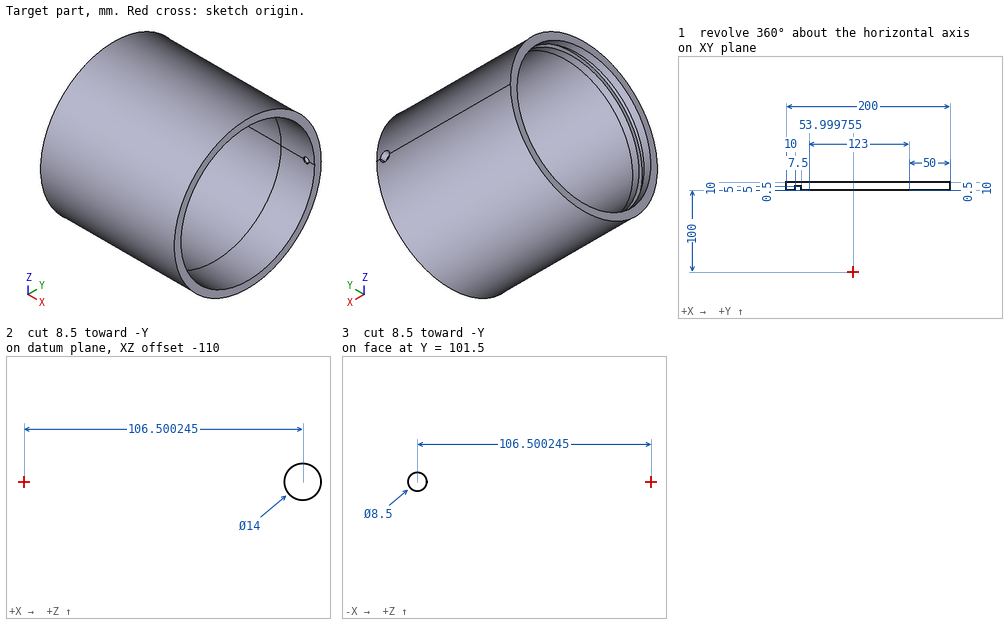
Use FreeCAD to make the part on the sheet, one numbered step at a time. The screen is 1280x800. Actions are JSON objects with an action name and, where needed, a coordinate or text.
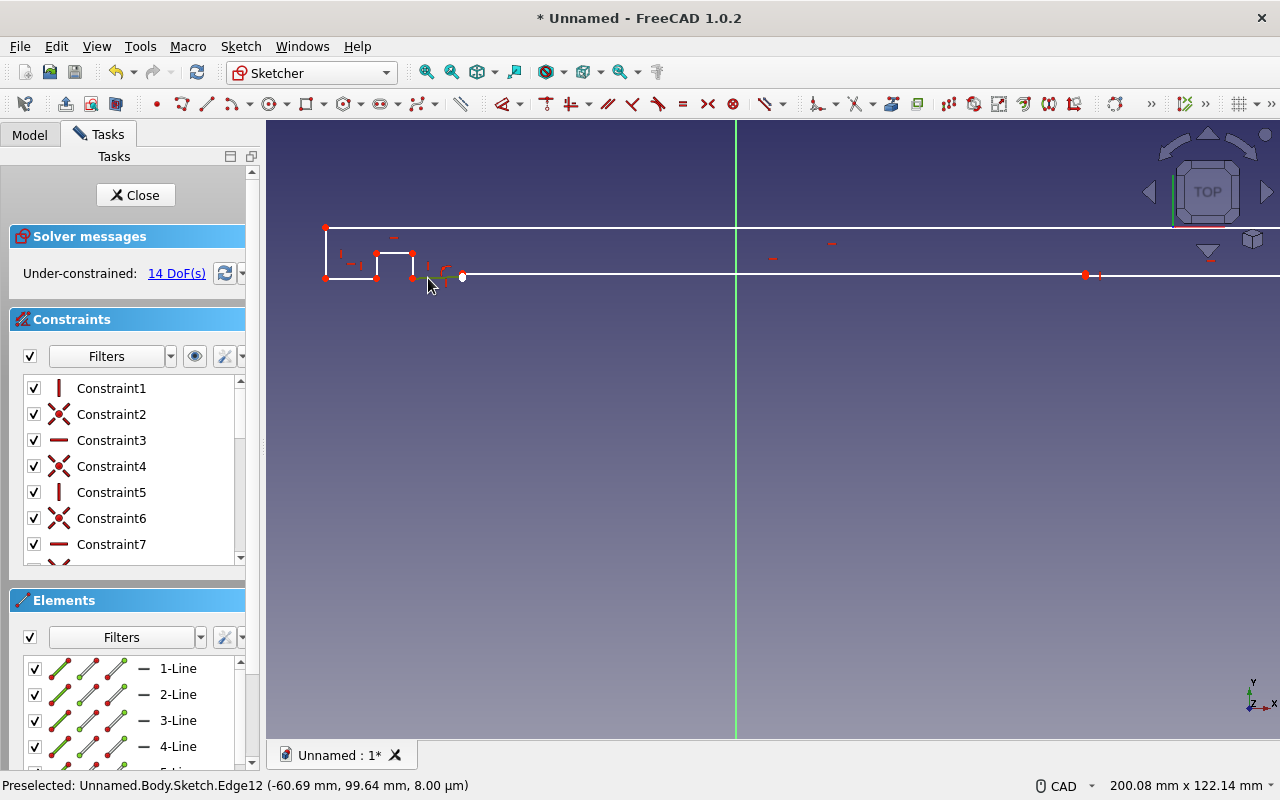
{"action": "key", "text": "h"}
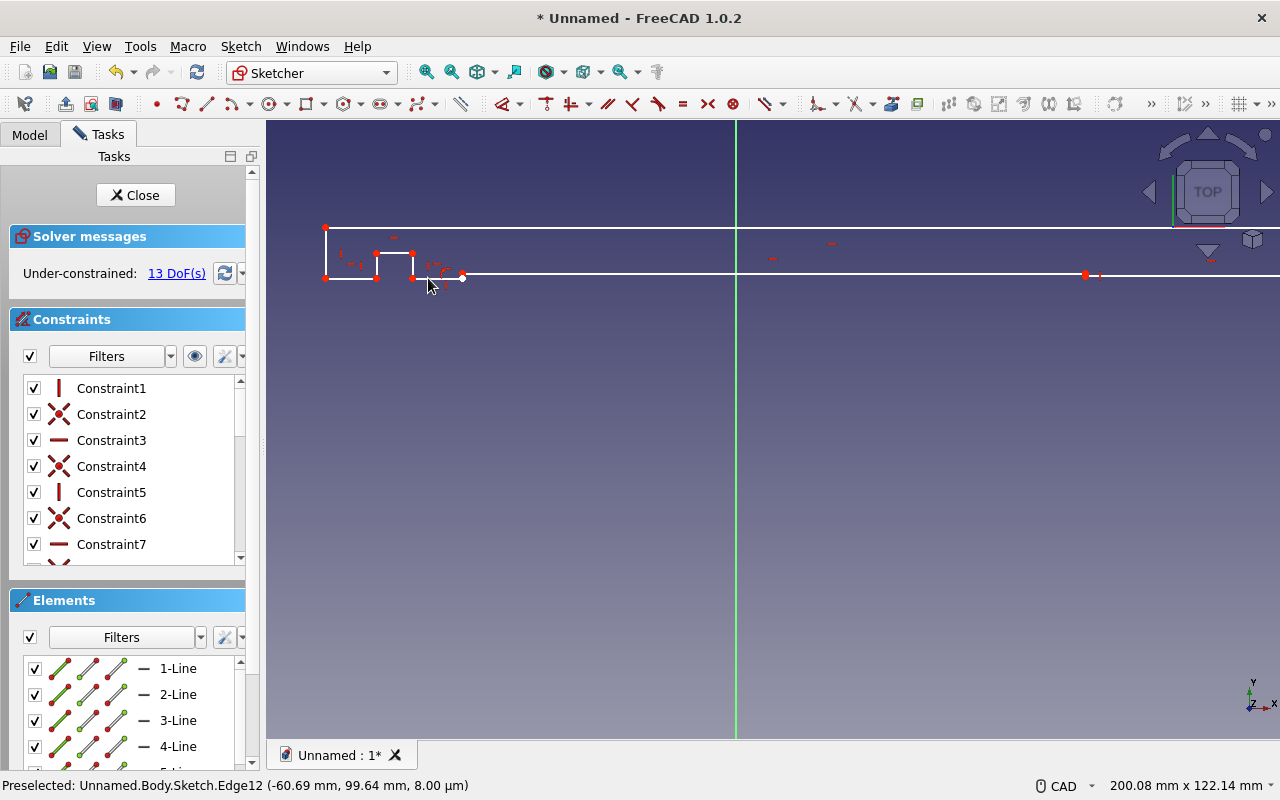
{"action": "left_click", "coordinate": [502, 104]}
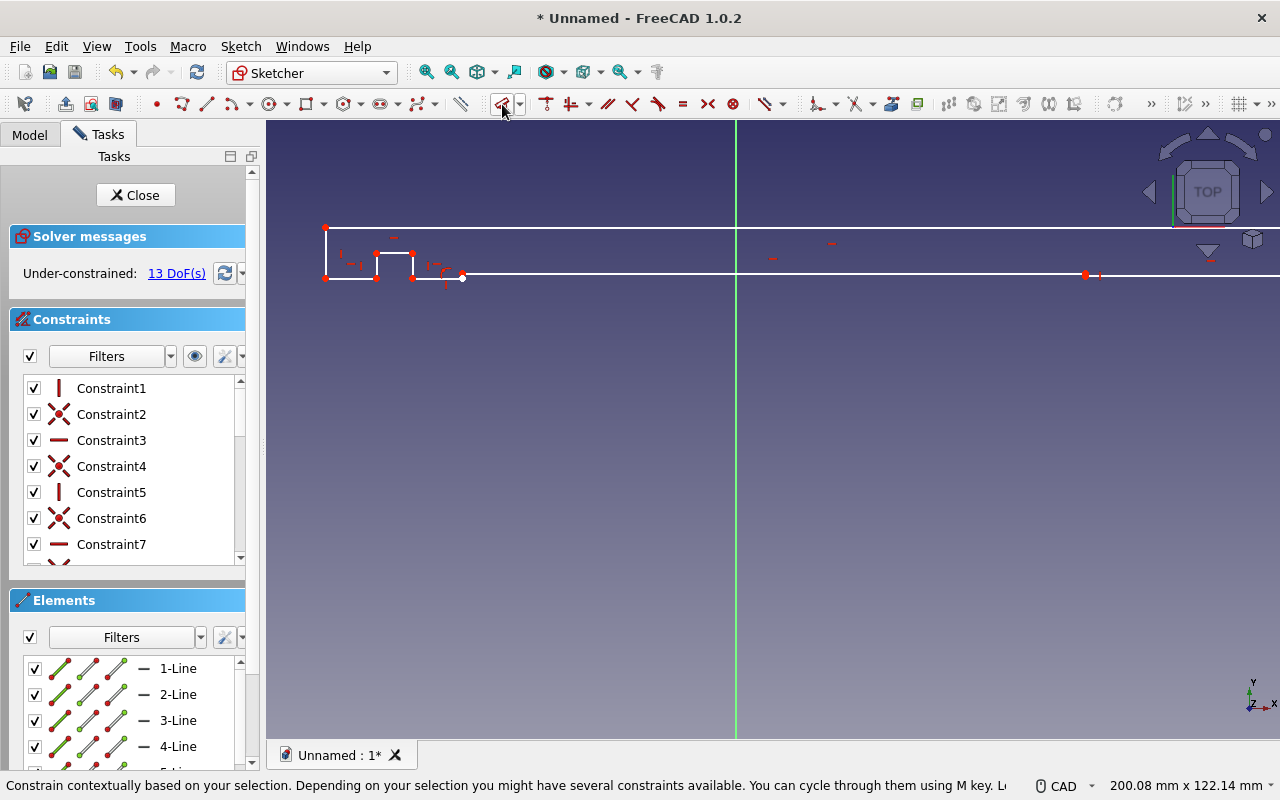
{"action": "scroll", "coordinate": [377, 268], "scroll_direction": "up", "scroll_amount": 3}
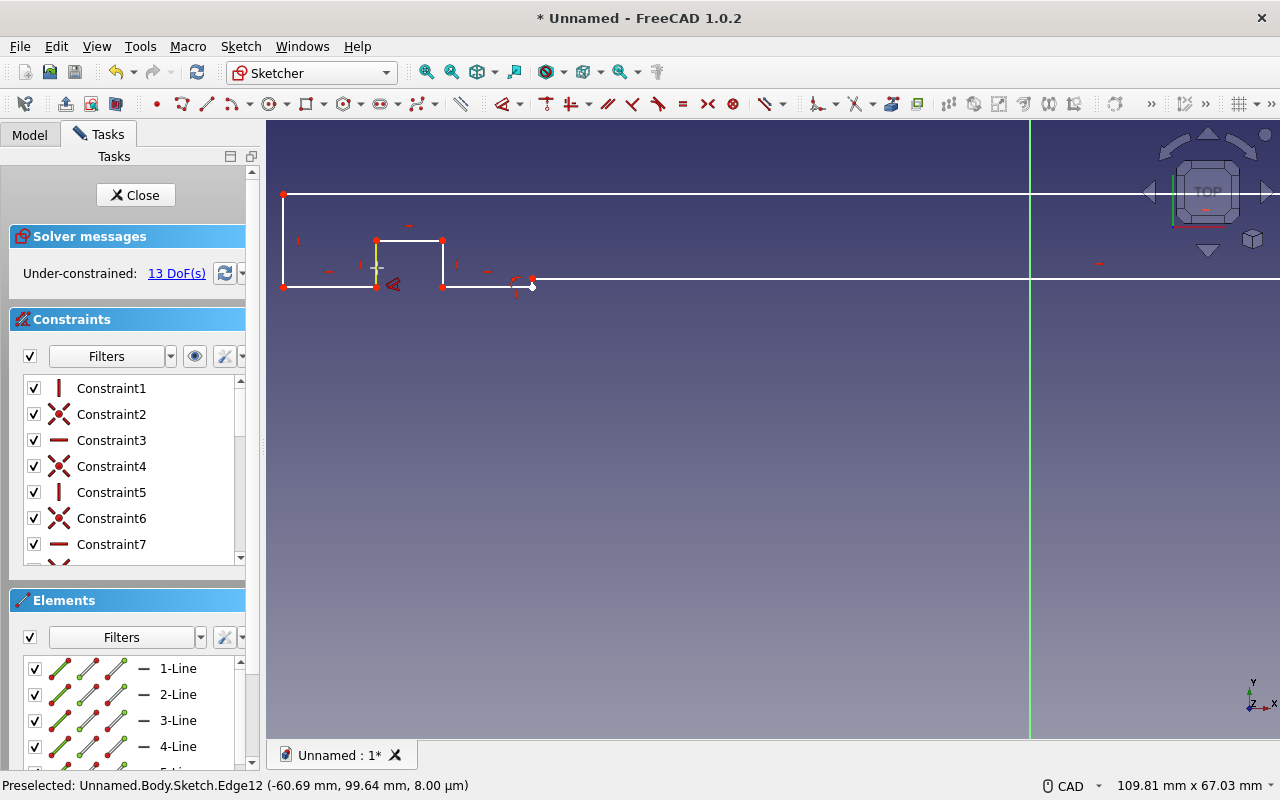
{"action": "left_click", "coordinate": [376, 269]}
{"action": "left_click", "coordinate": [342, 264]}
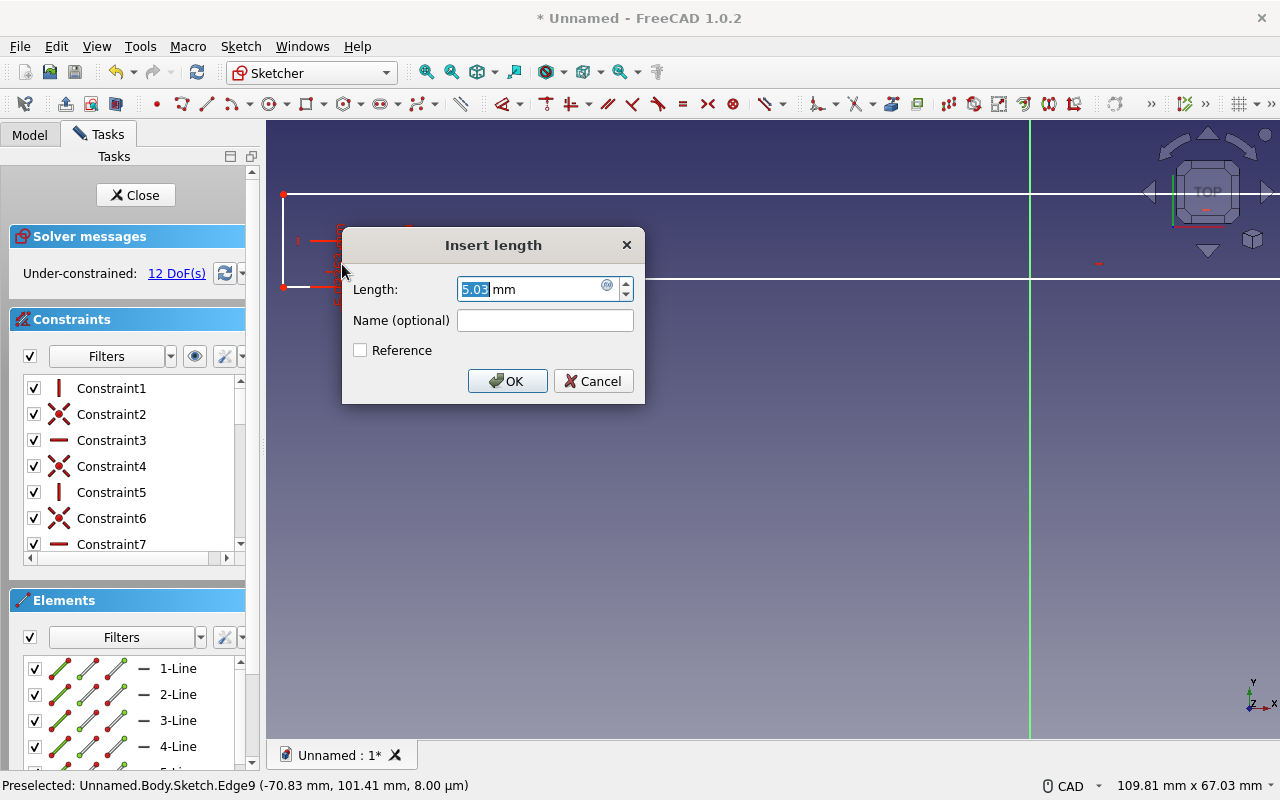
{"action": "type", "text": "5"}
{"action": "key", "text": "Return"}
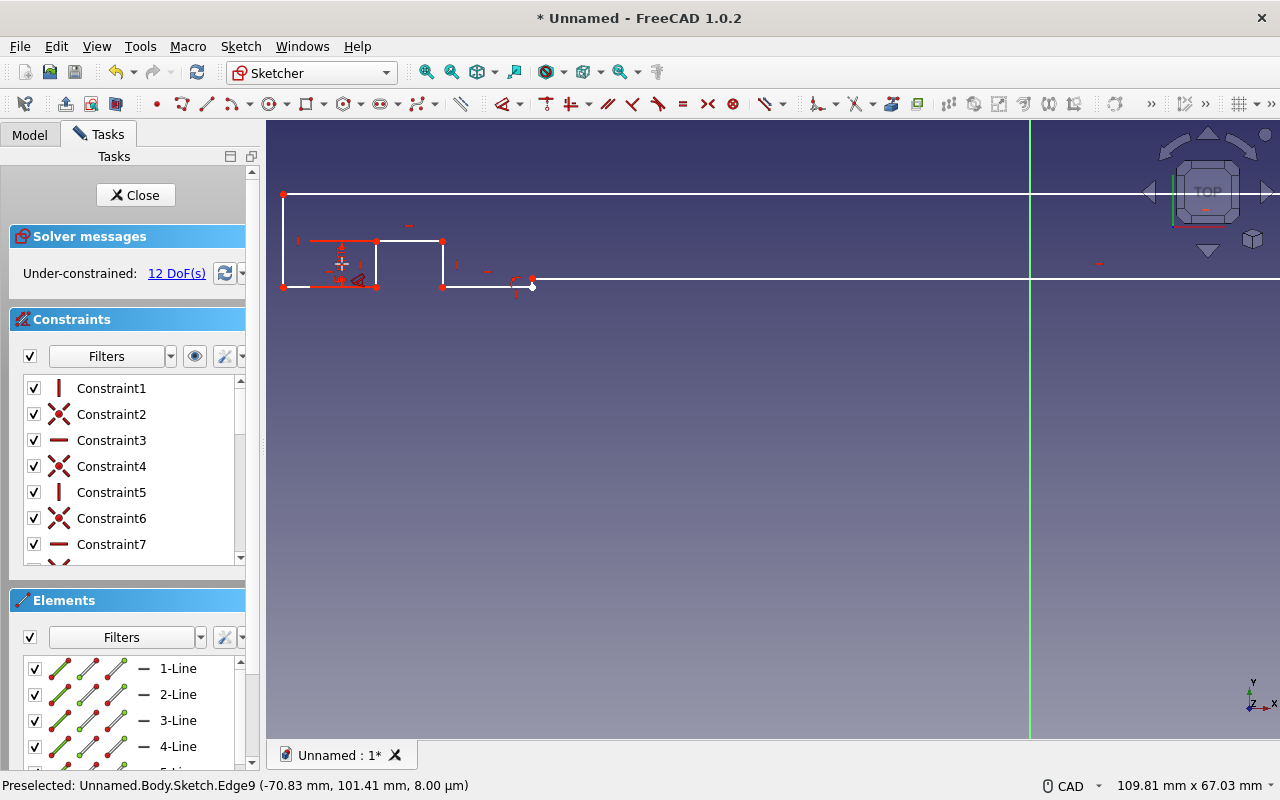
{"action": "left_click", "coordinate": [443, 255]}
{"action": "left_click", "coordinate": [477, 264]}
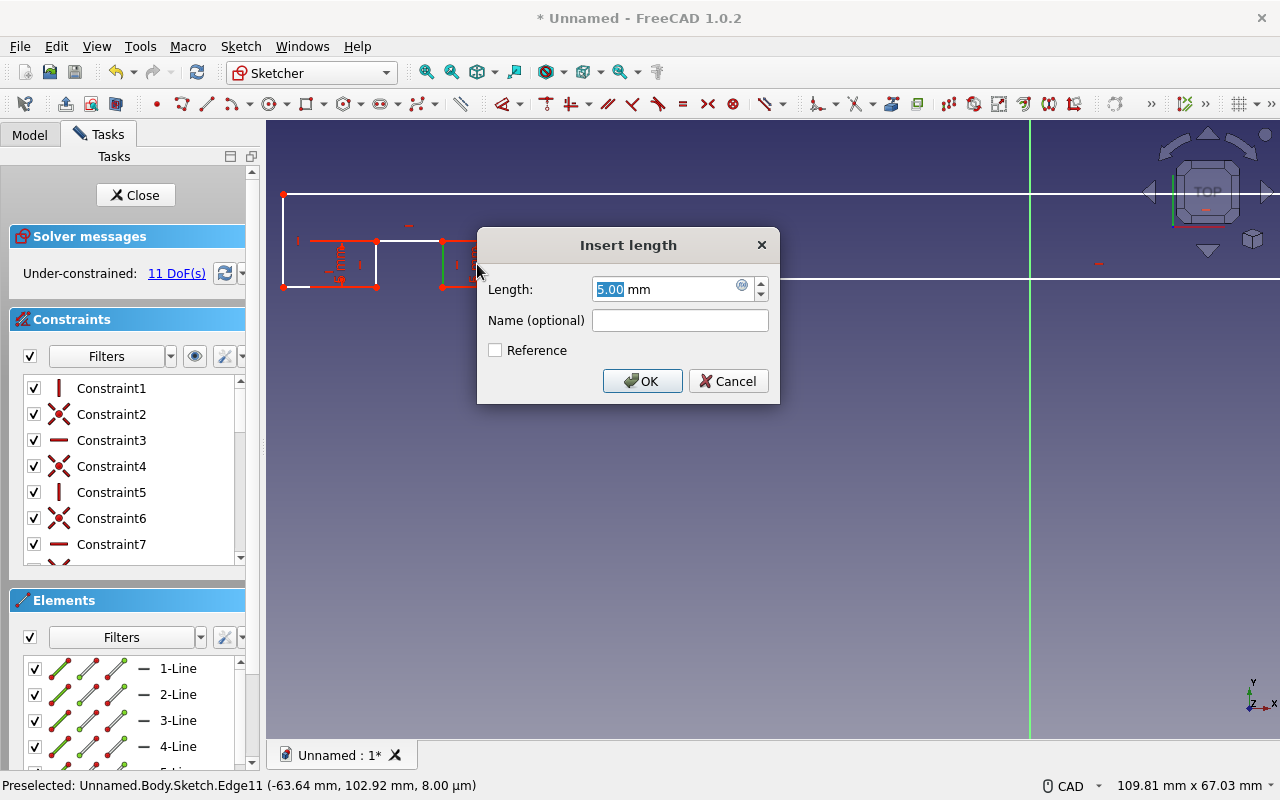
{"action": "type", "text": "5"}
{"action": "key", "text": "Return"}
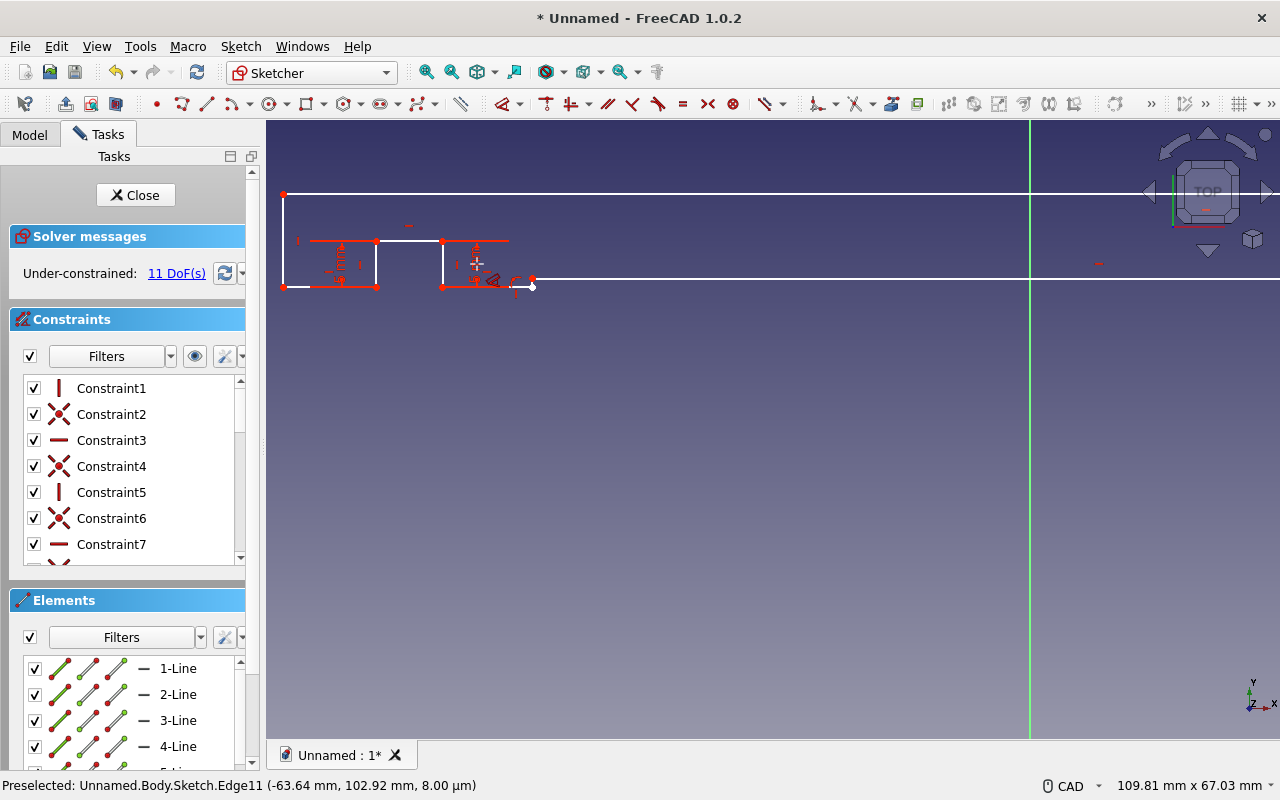
{"action": "scroll", "coordinate": [488, 314], "scroll_direction": "down", "scroll_amount": 6}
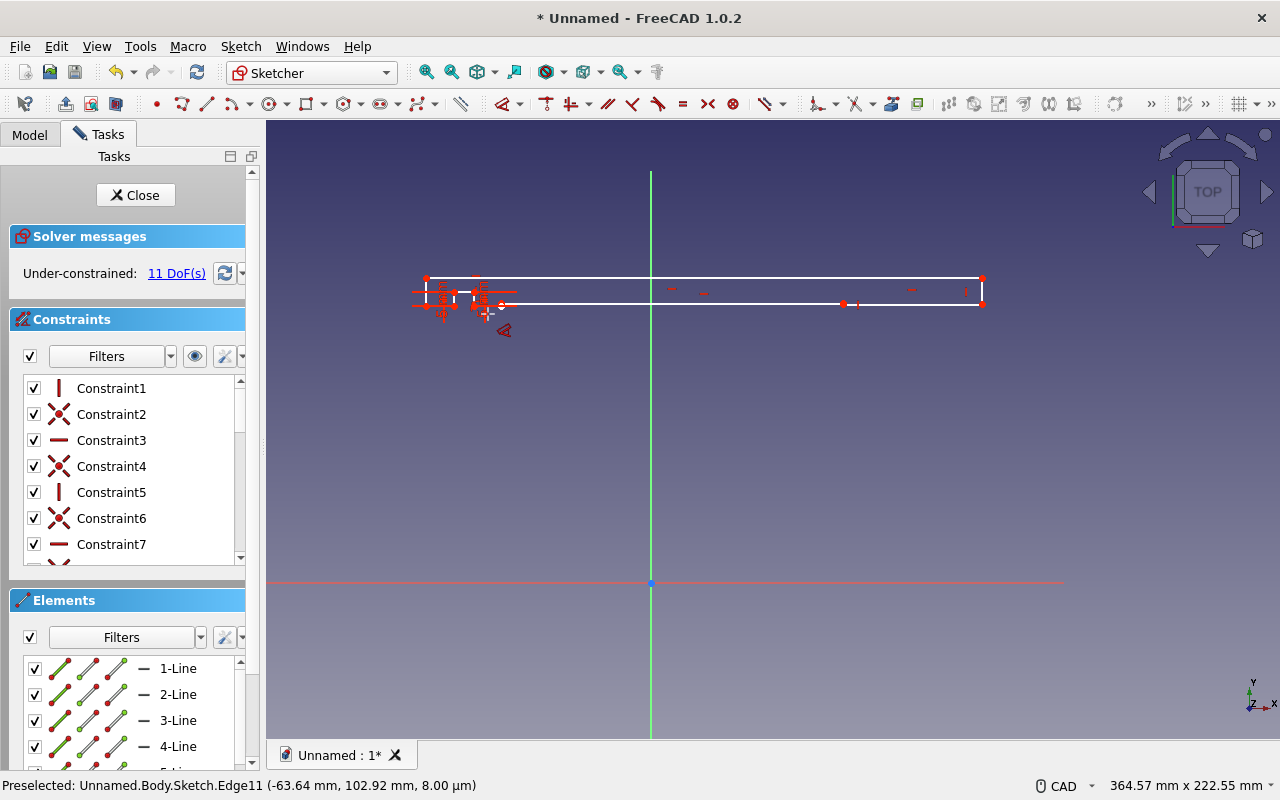
{"action": "left_click", "coordinate": [885, 305]}
{"action": "left_click", "coordinate": [913, 339]}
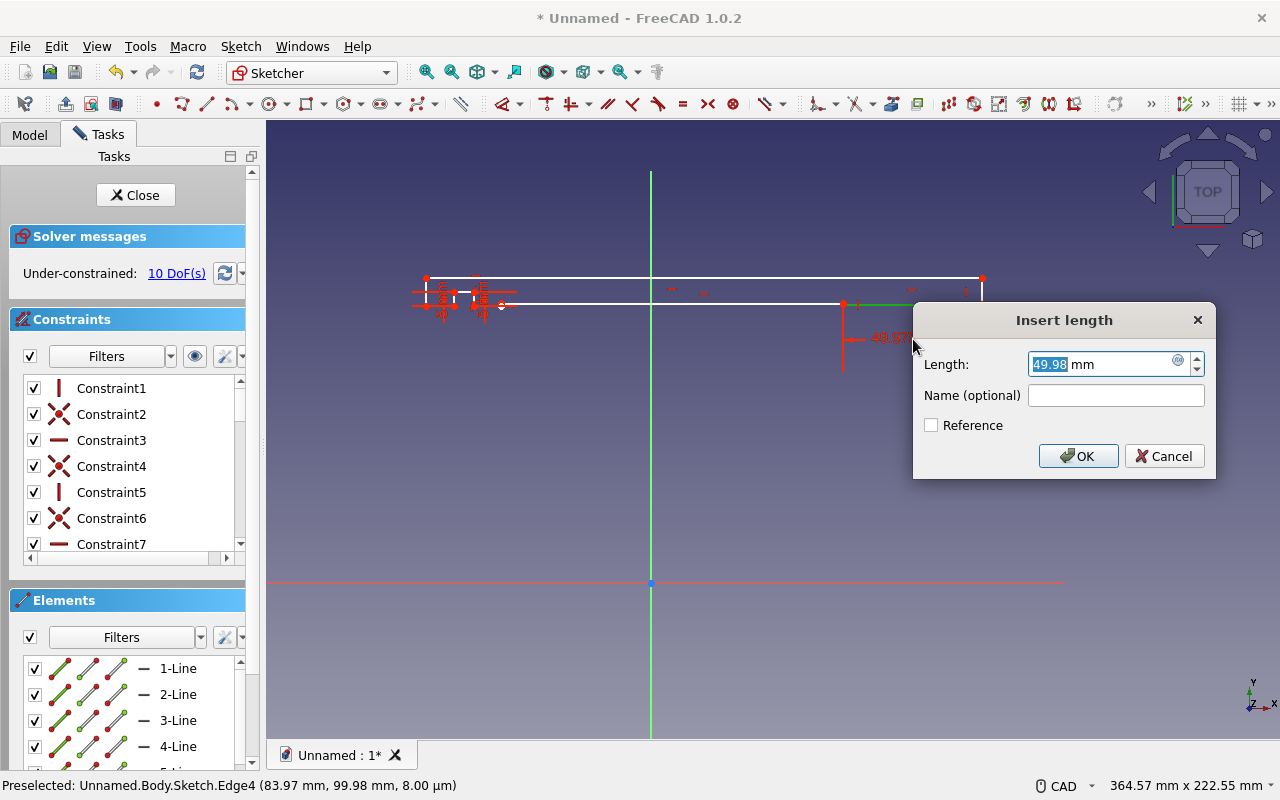
{"action": "type", "text": "50"}
{"action": "key", "text": "Return"}